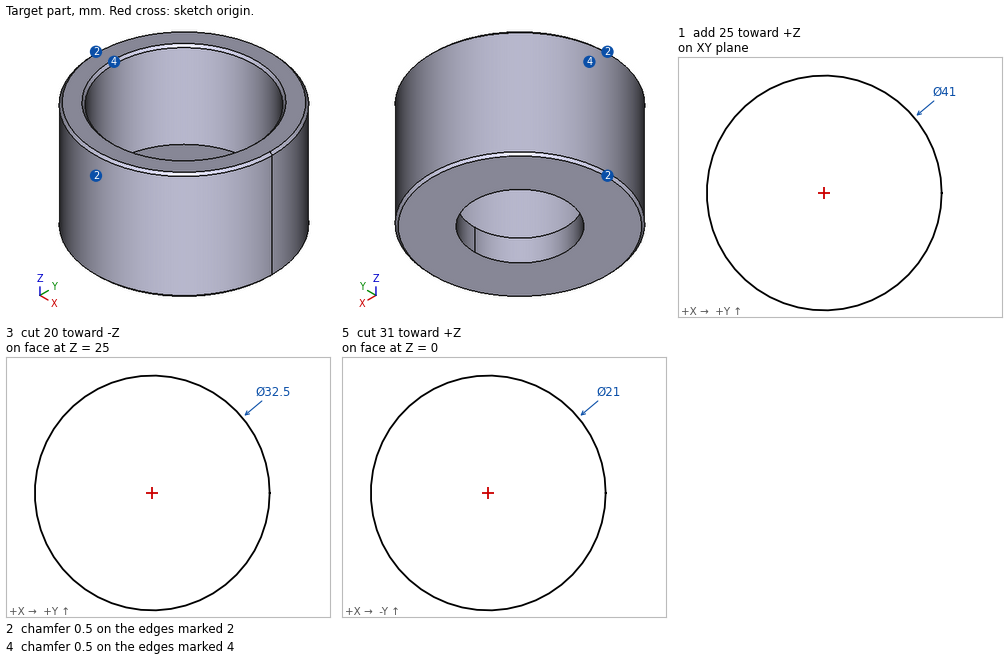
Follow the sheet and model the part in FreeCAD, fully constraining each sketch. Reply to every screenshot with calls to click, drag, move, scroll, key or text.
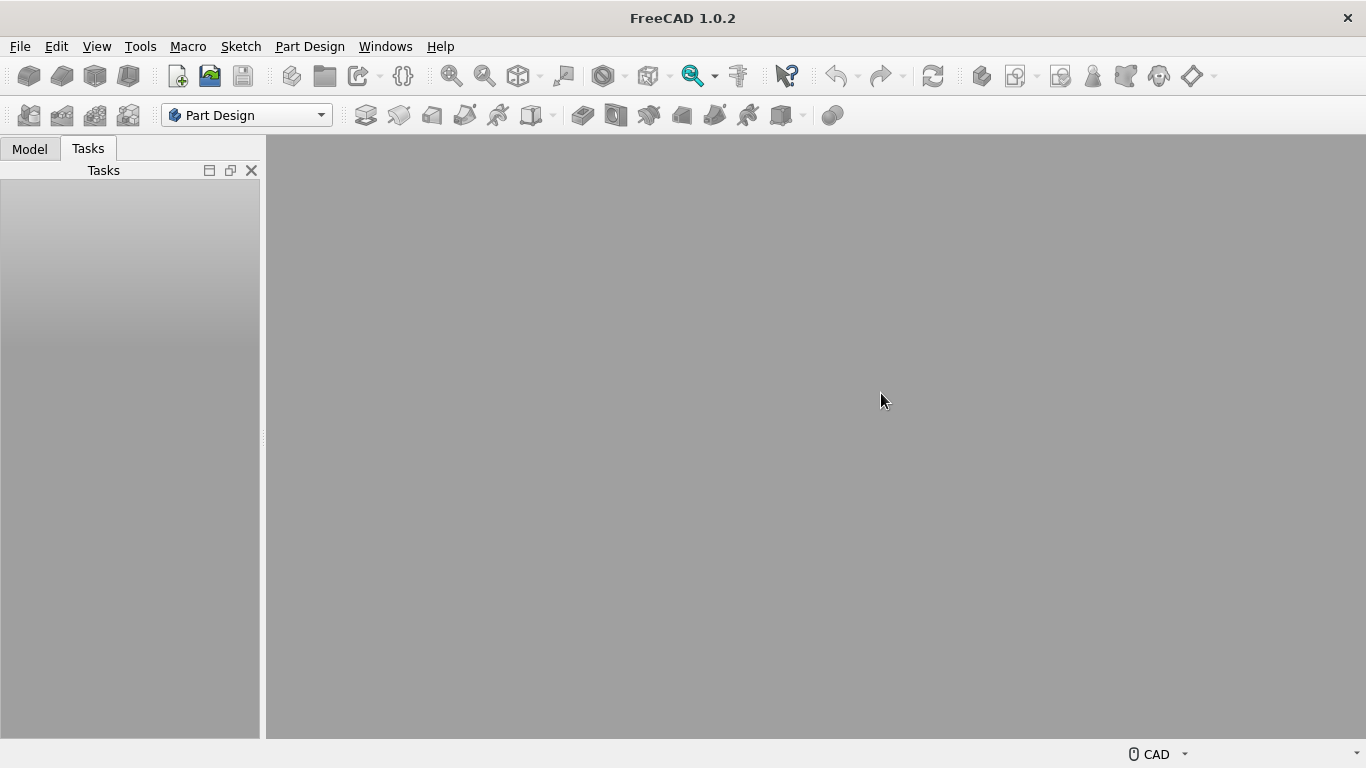
click(177, 76)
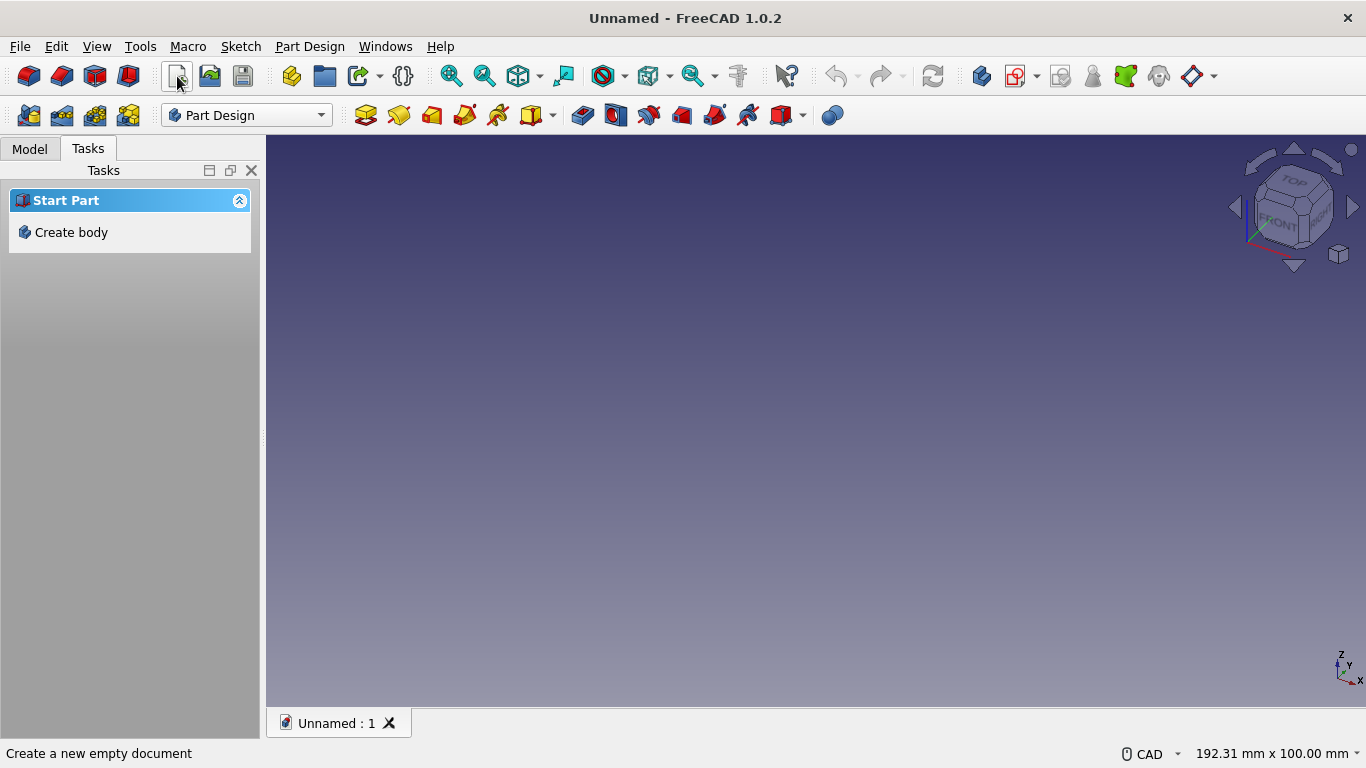
click(1014, 76)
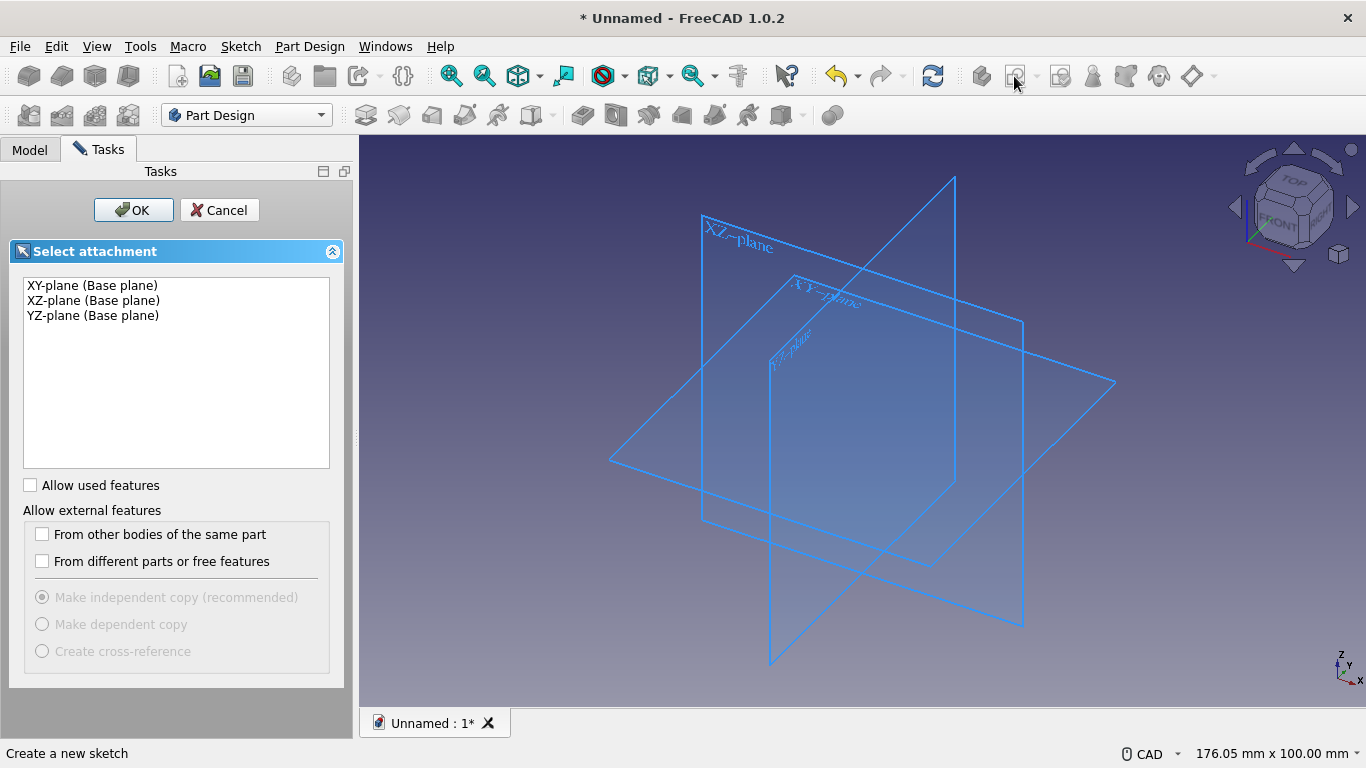
click(84, 286)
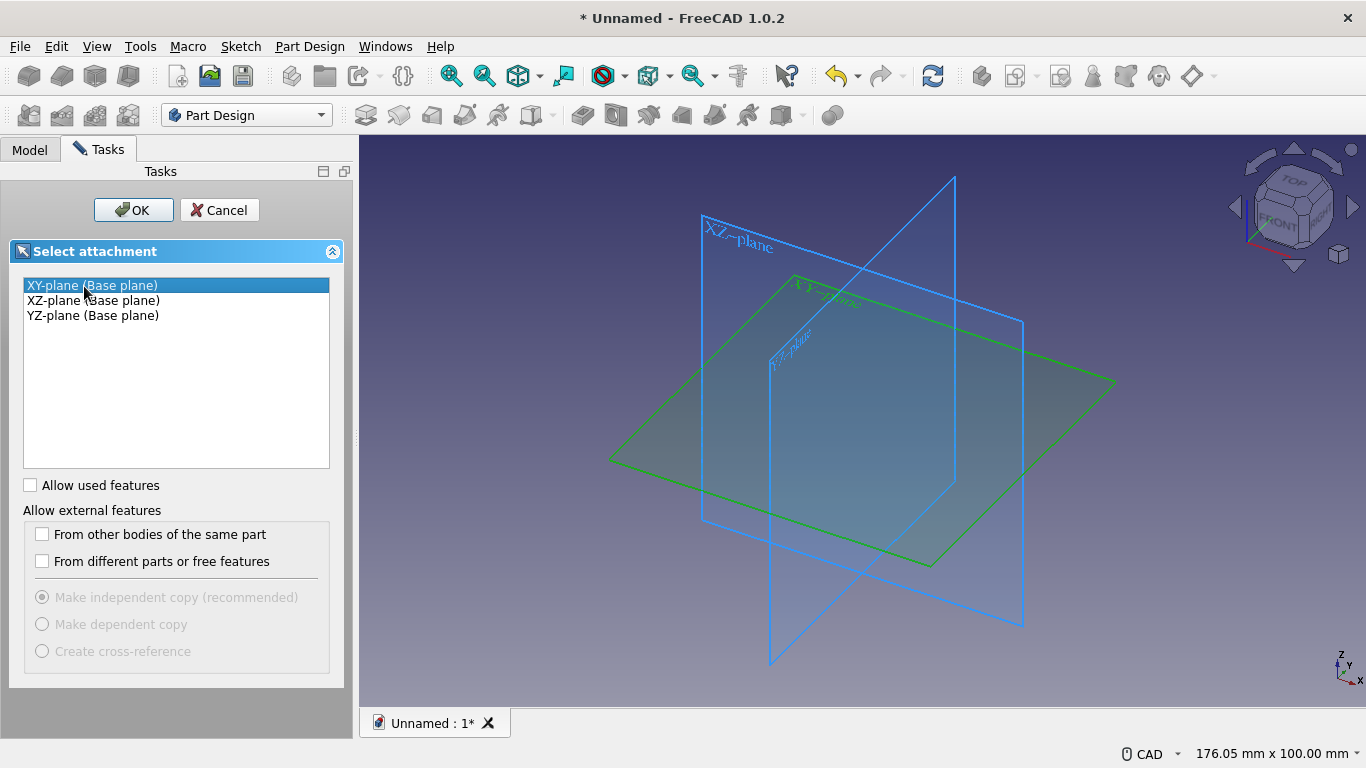
click(134, 210)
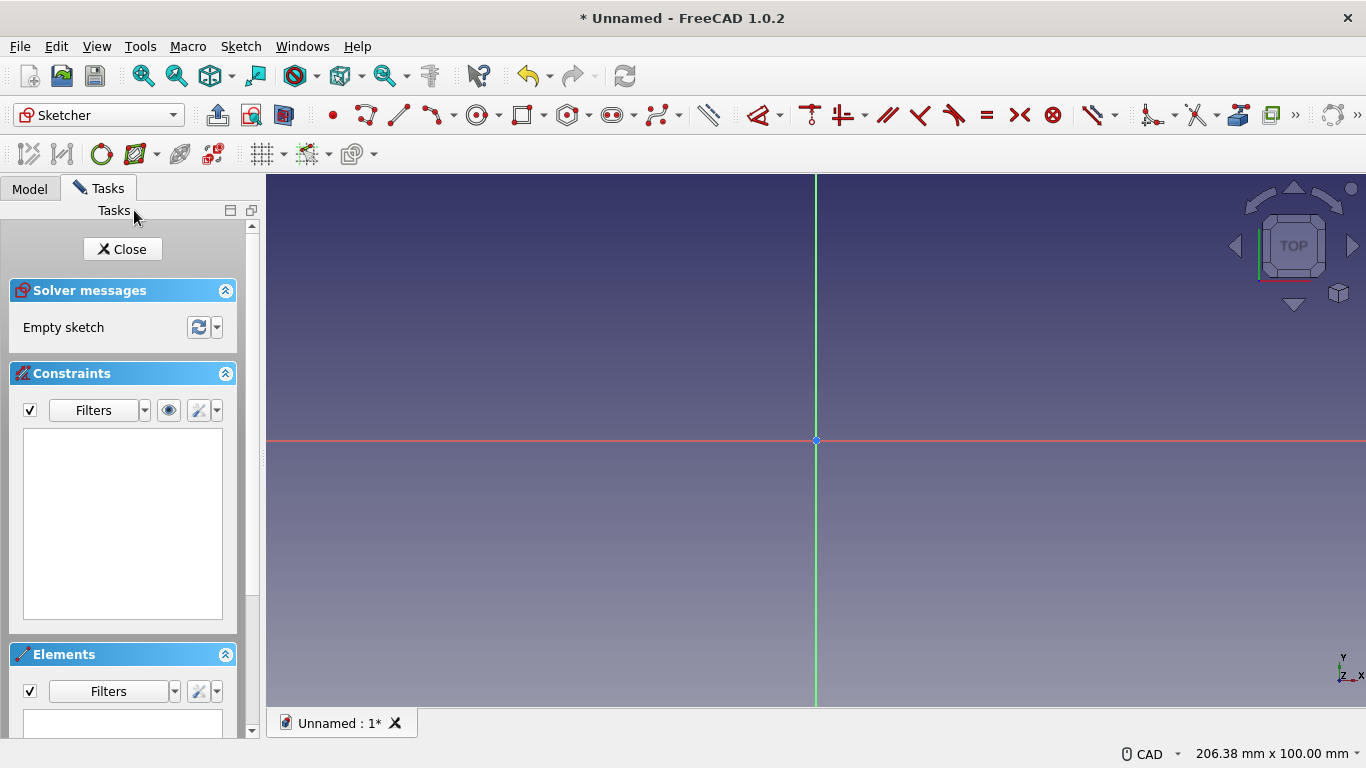
scroll(955, 440, up, 2)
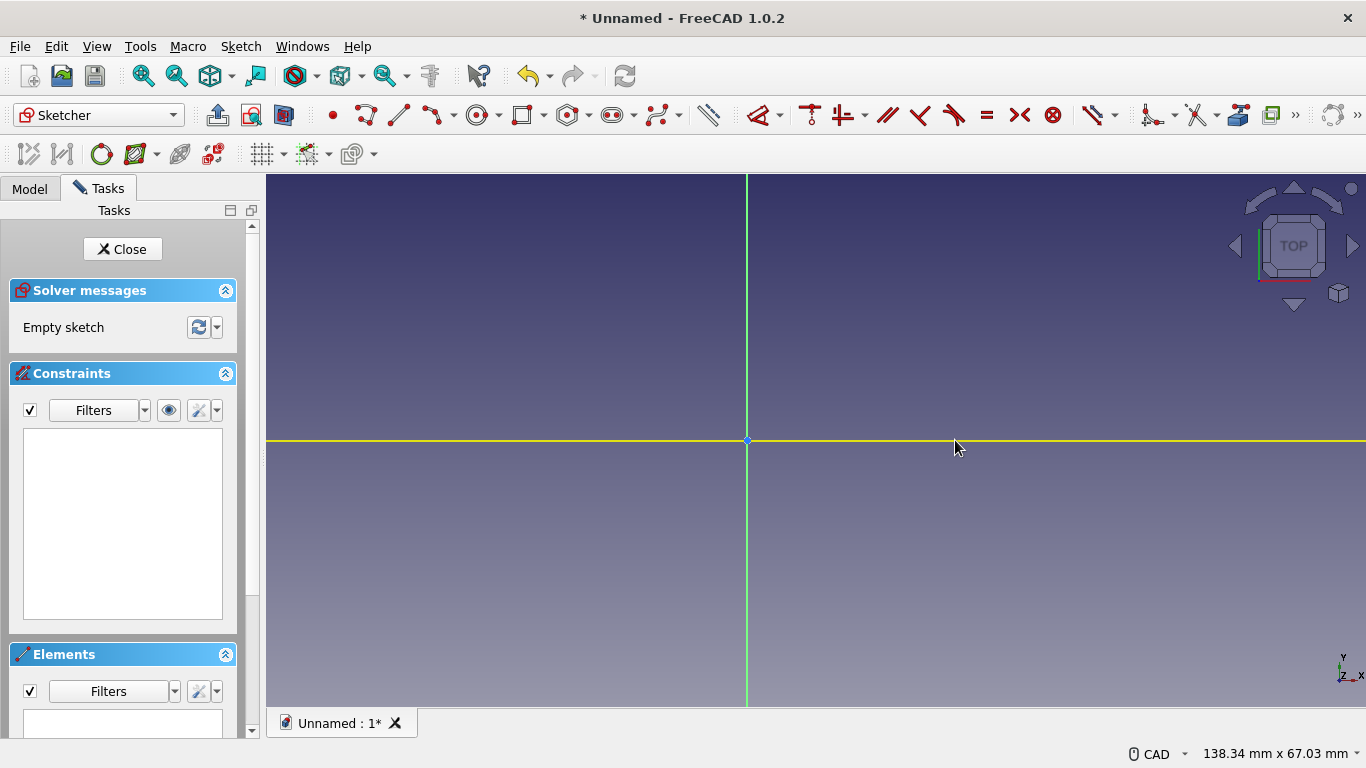
click(476, 116)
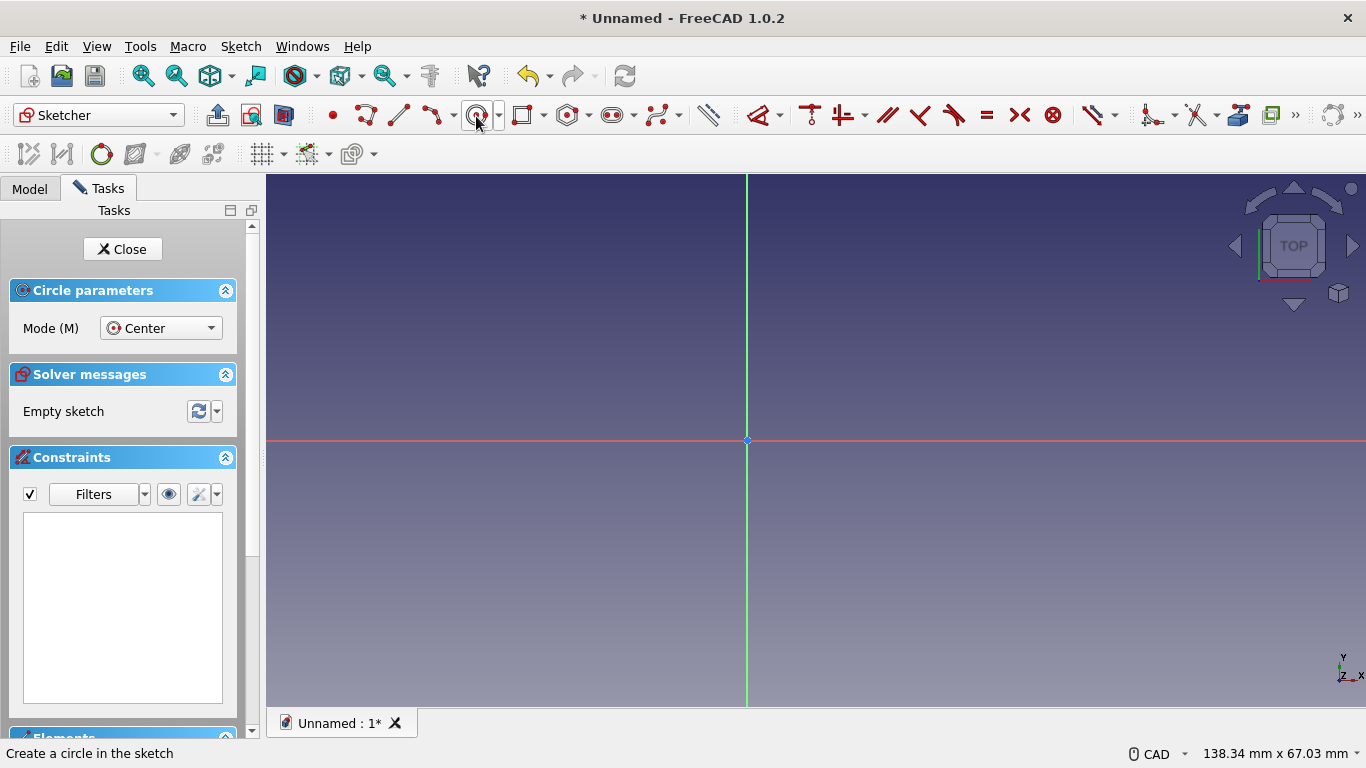
click(747, 440)
move(863, 325)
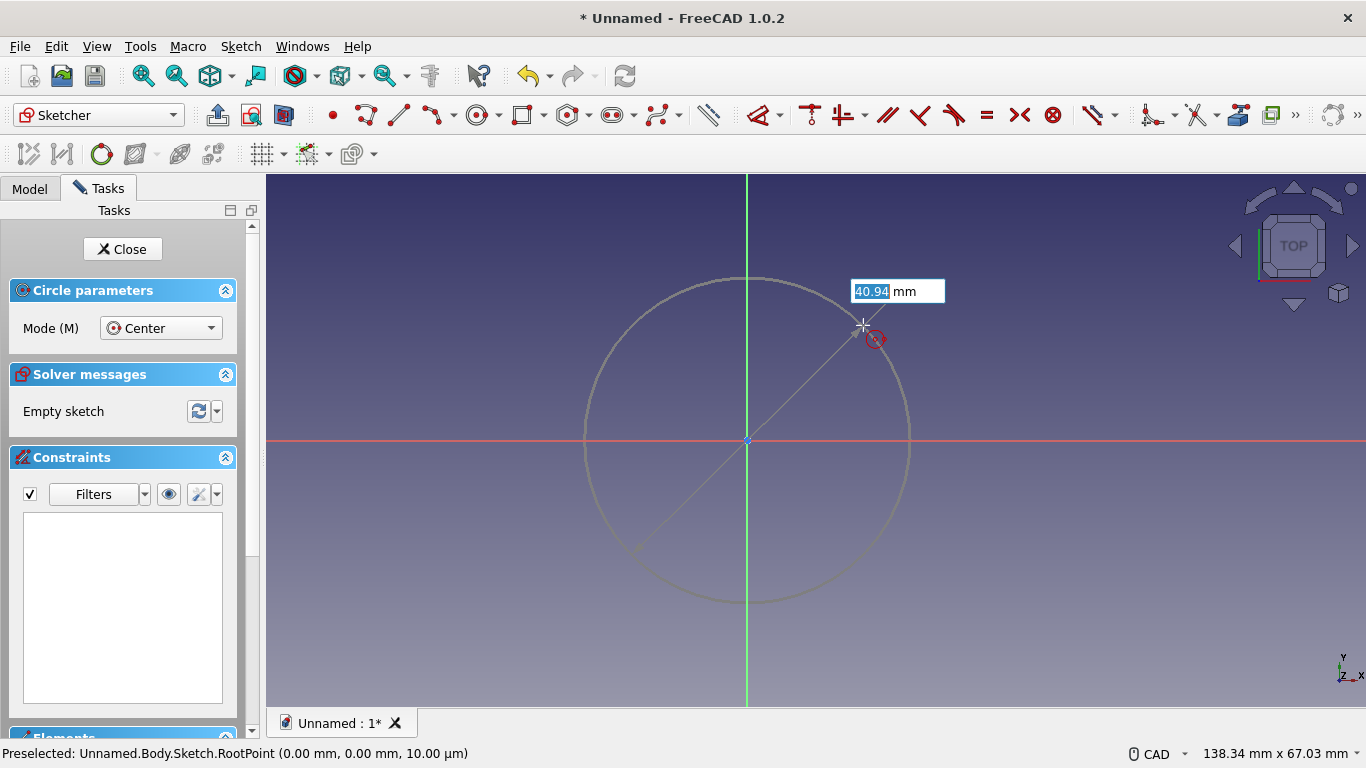
text(41)
key(Return)
key(Escape)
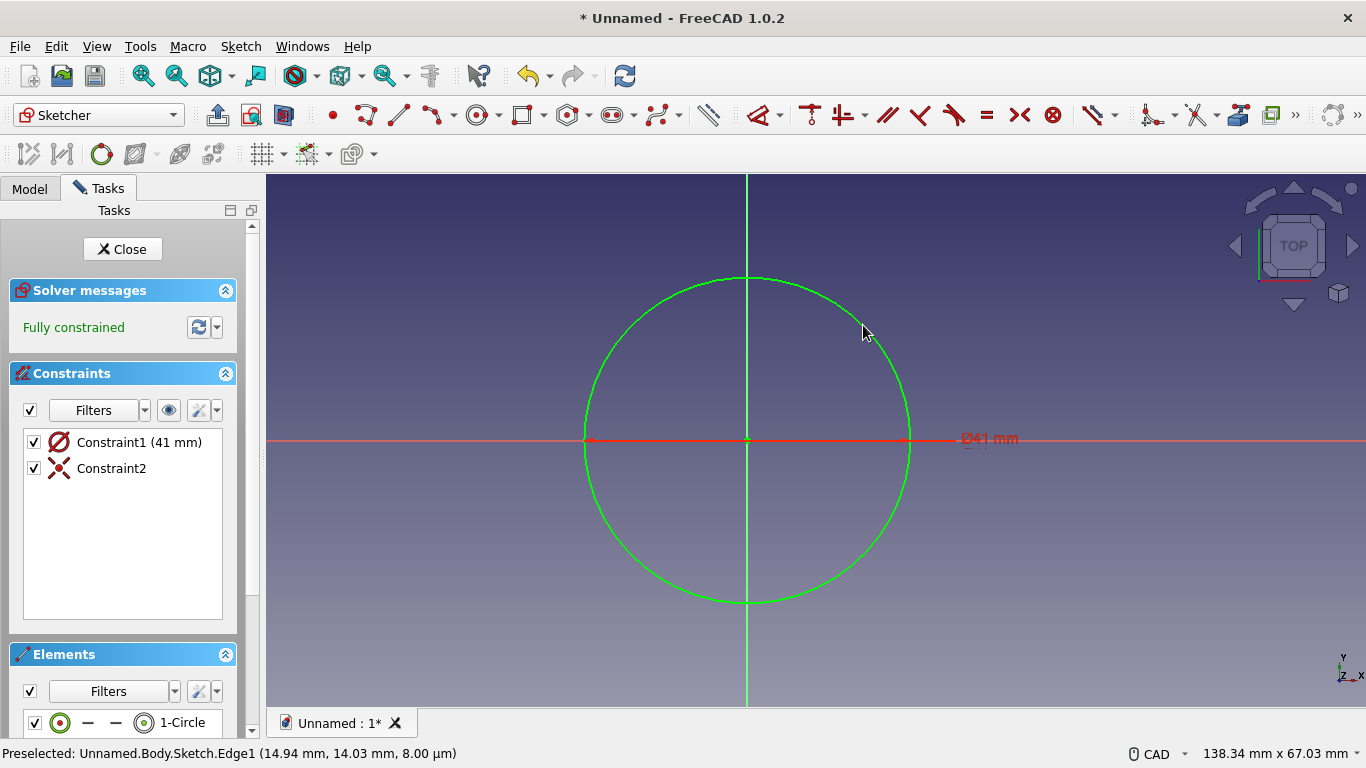
click(123, 249)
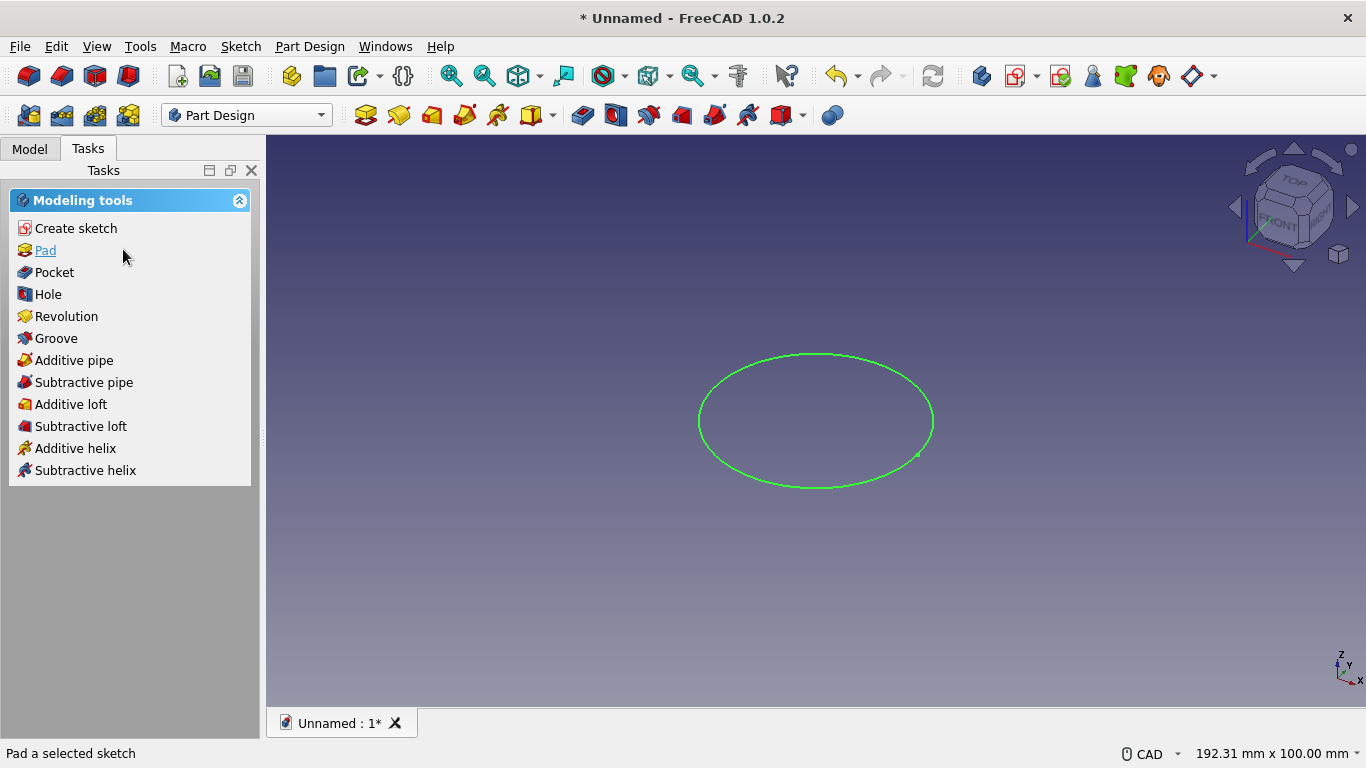
click(366, 116)